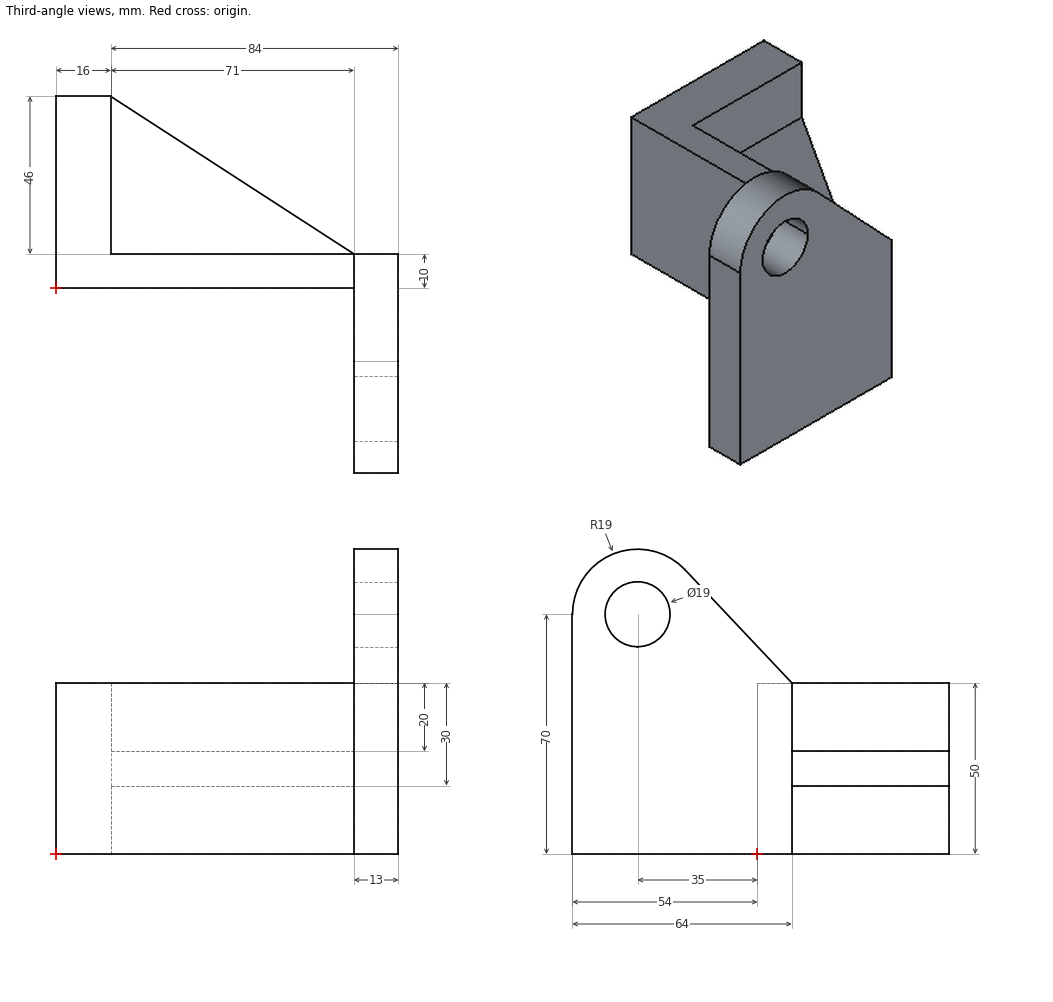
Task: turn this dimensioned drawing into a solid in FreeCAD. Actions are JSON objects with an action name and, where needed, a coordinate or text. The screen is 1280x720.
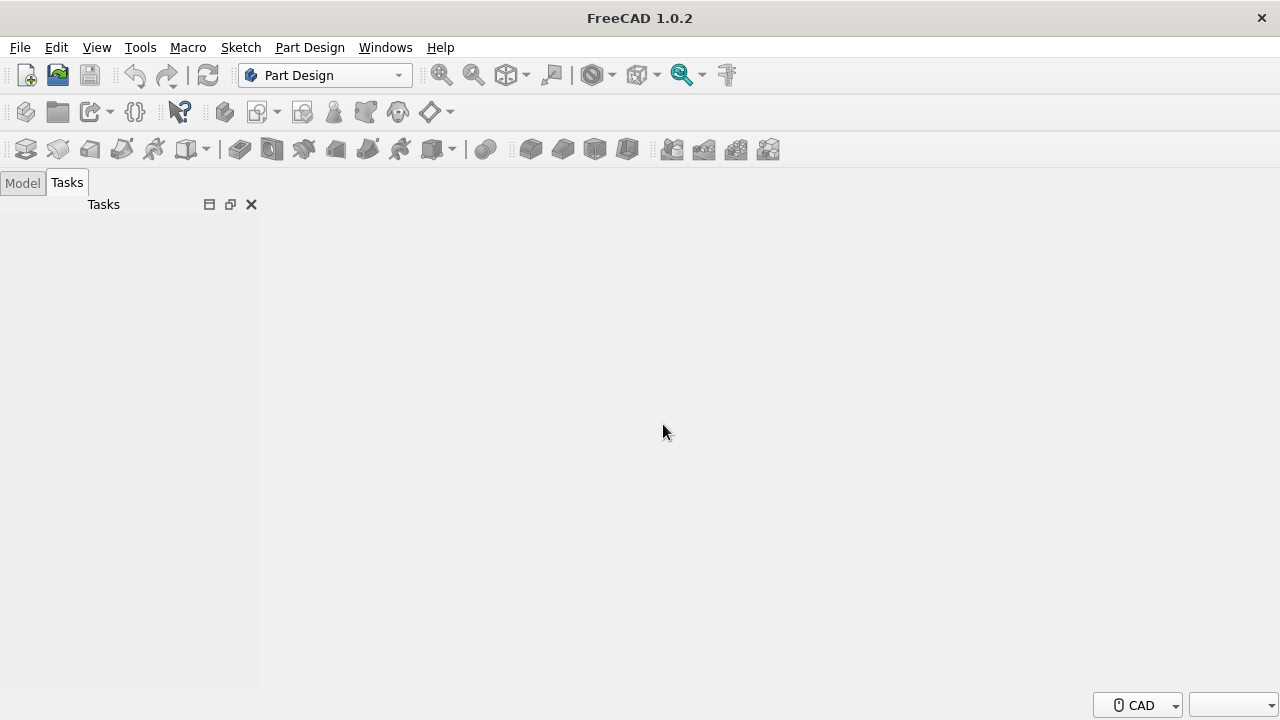
{"action": "key", "text": "ctrl+n"}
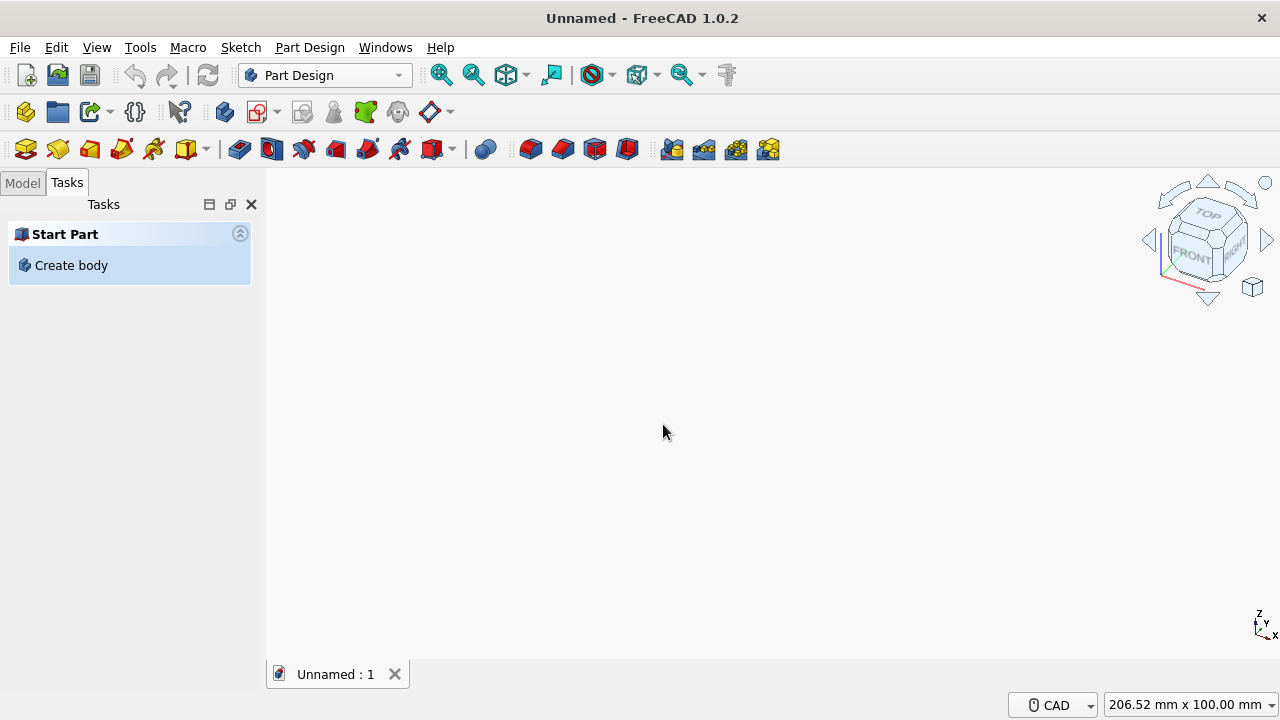
{"action": "left_click", "coordinate": [258, 112]}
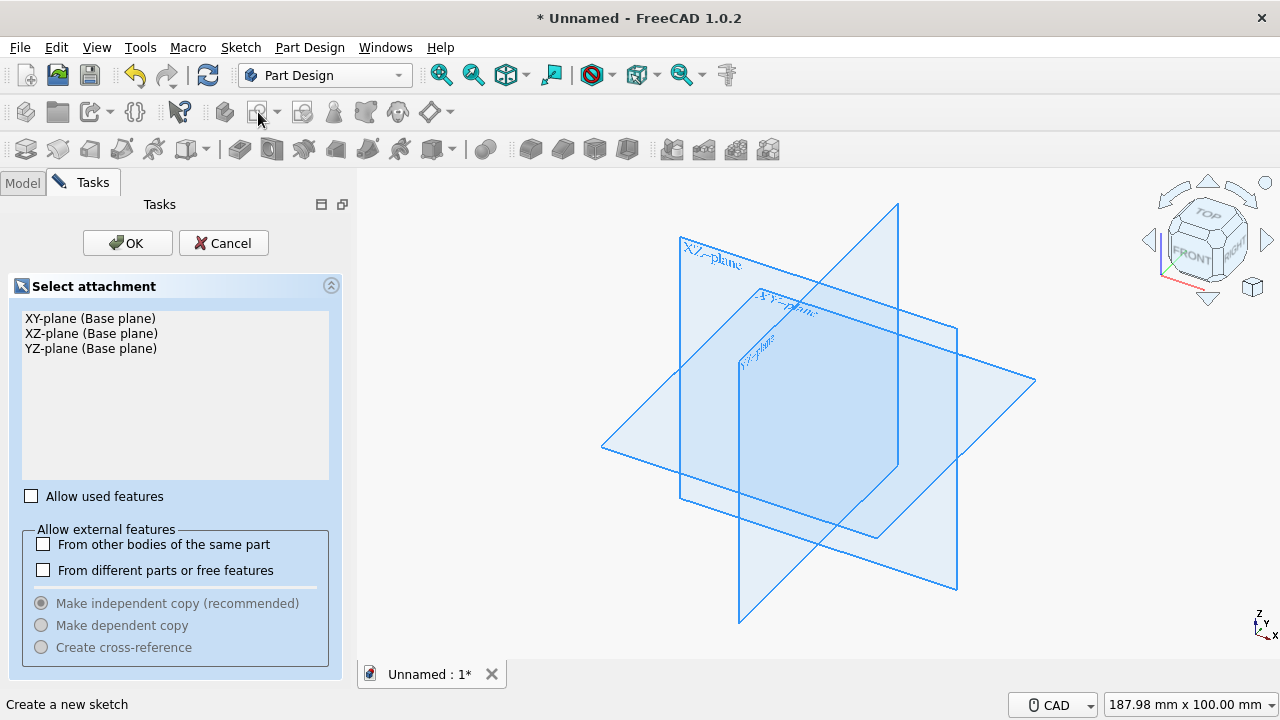
{"action": "left_click", "coordinate": [82, 318]}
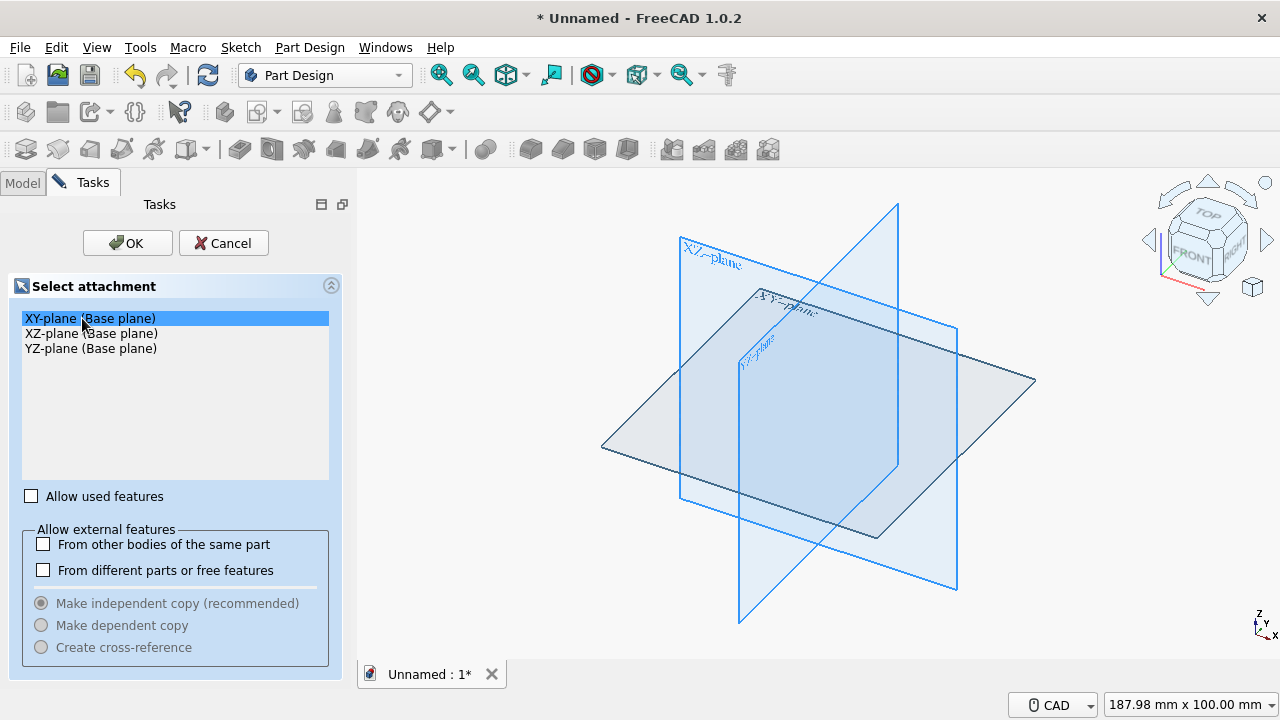
{"action": "left_click", "coordinate": [128, 243]}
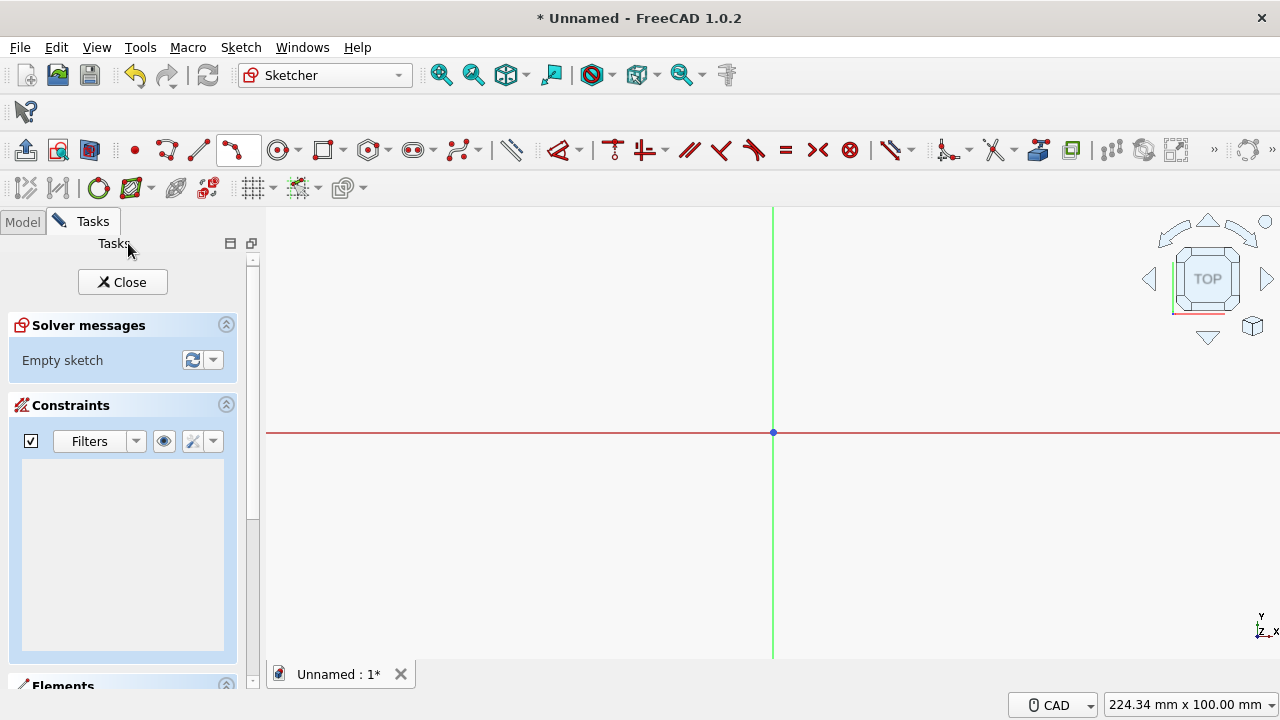
{"action": "scroll", "coordinate": [294, 631], "scroll_direction": "down", "scroll_amount": 1}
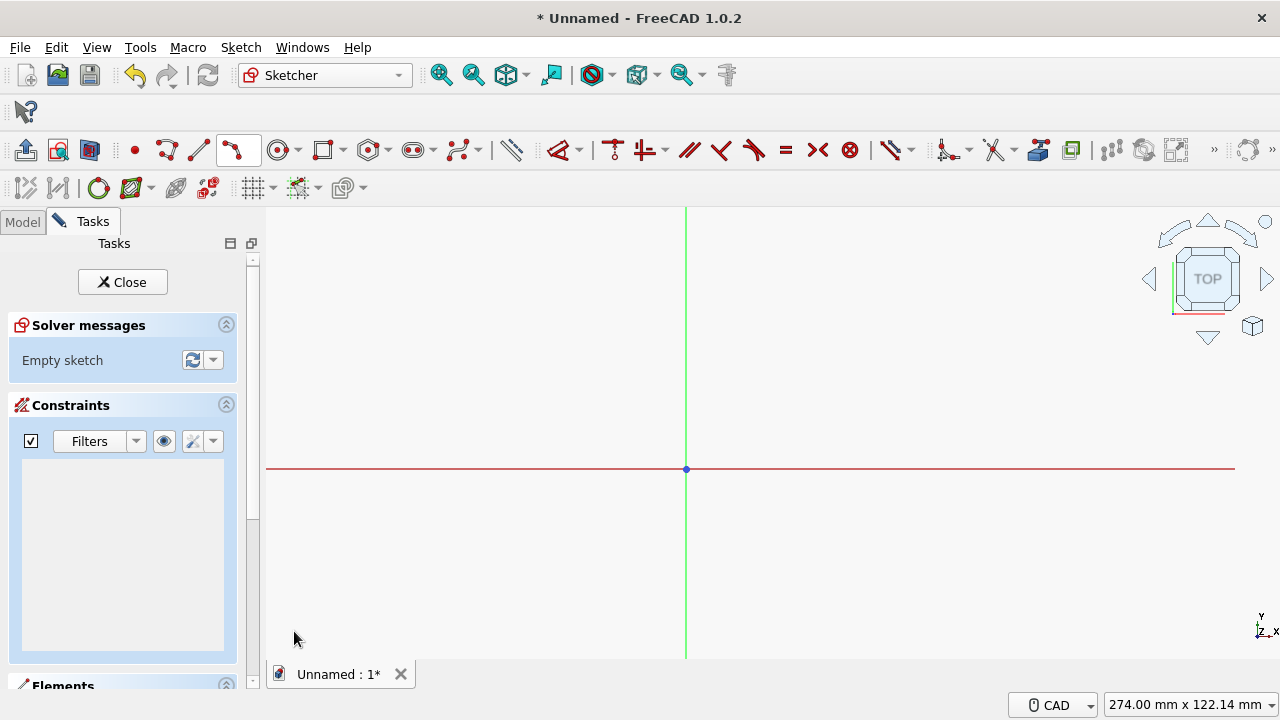
{"action": "key", "text": "g m"}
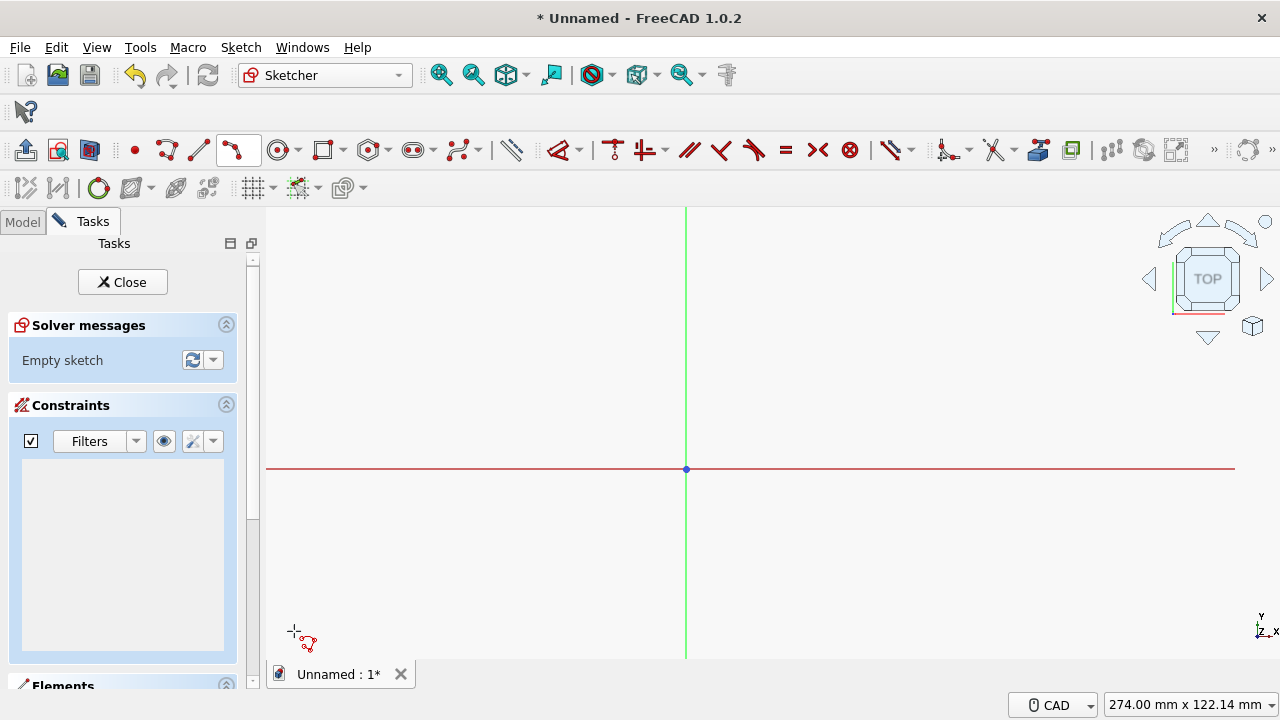
{"action": "left_click", "coordinate": [686, 469]}
{"action": "left_click", "coordinate": [1056, 460]}
{"action": "left_click", "coordinate": [1056, 432]}
{"action": "left_click", "coordinate": [745, 432]}
{"action": "left_click", "coordinate": [745, 262]}
{"action": "left_click", "coordinate": [695, 262]}
{"action": "left_click", "coordinate": [686, 469]}
{"action": "key", "text": "Escape"}
{"action": "key", "text": "Escape"}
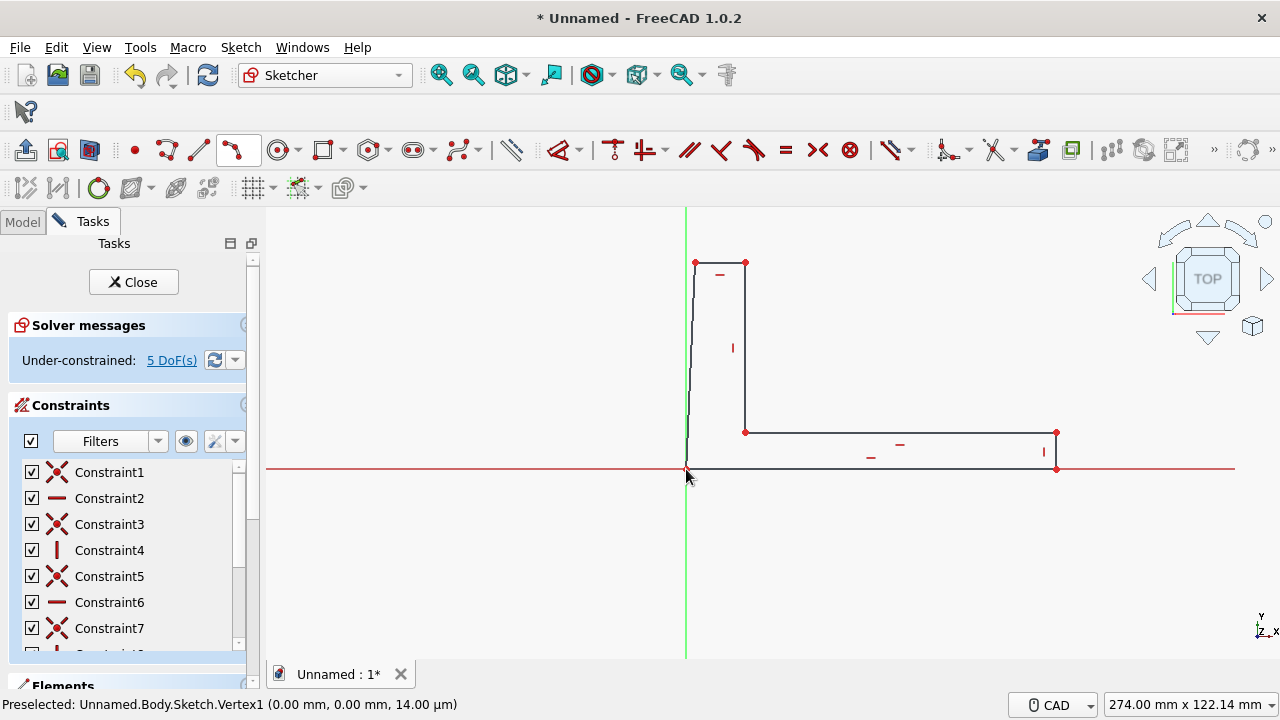
{"action": "left_click", "coordinate": [689, 407]}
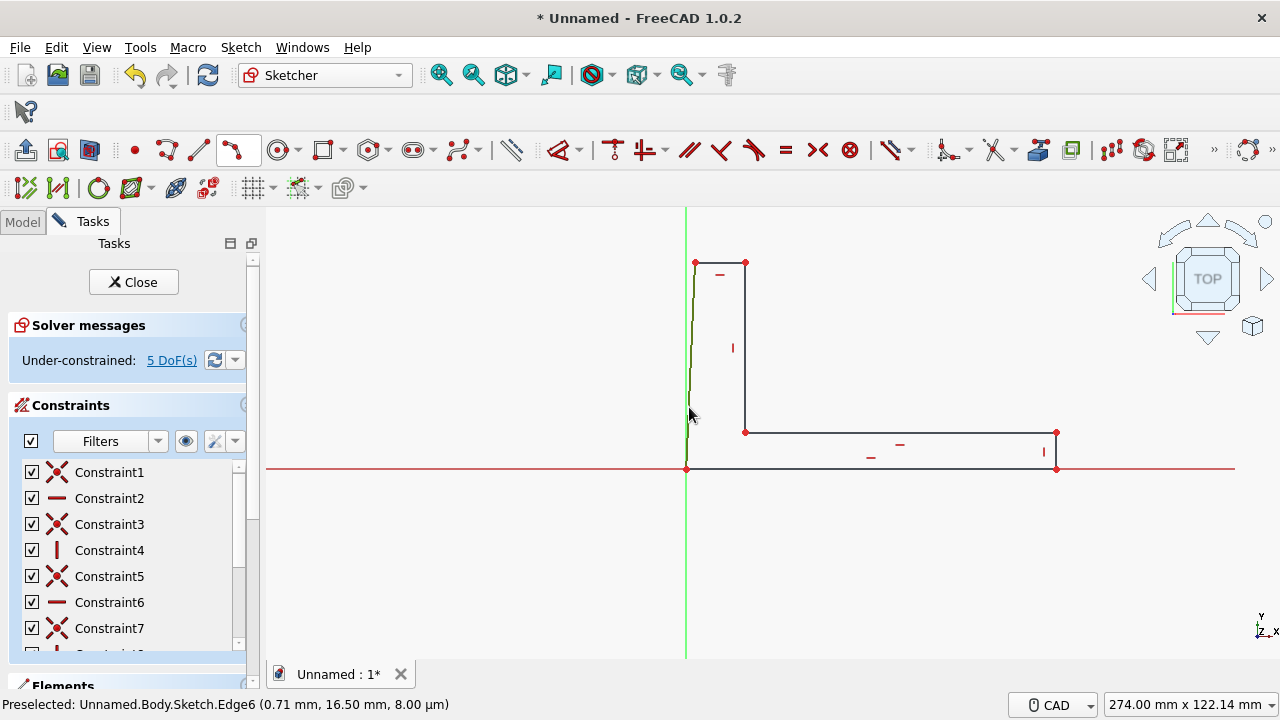
{"action": "left_click", "coordinate": [668, 150]}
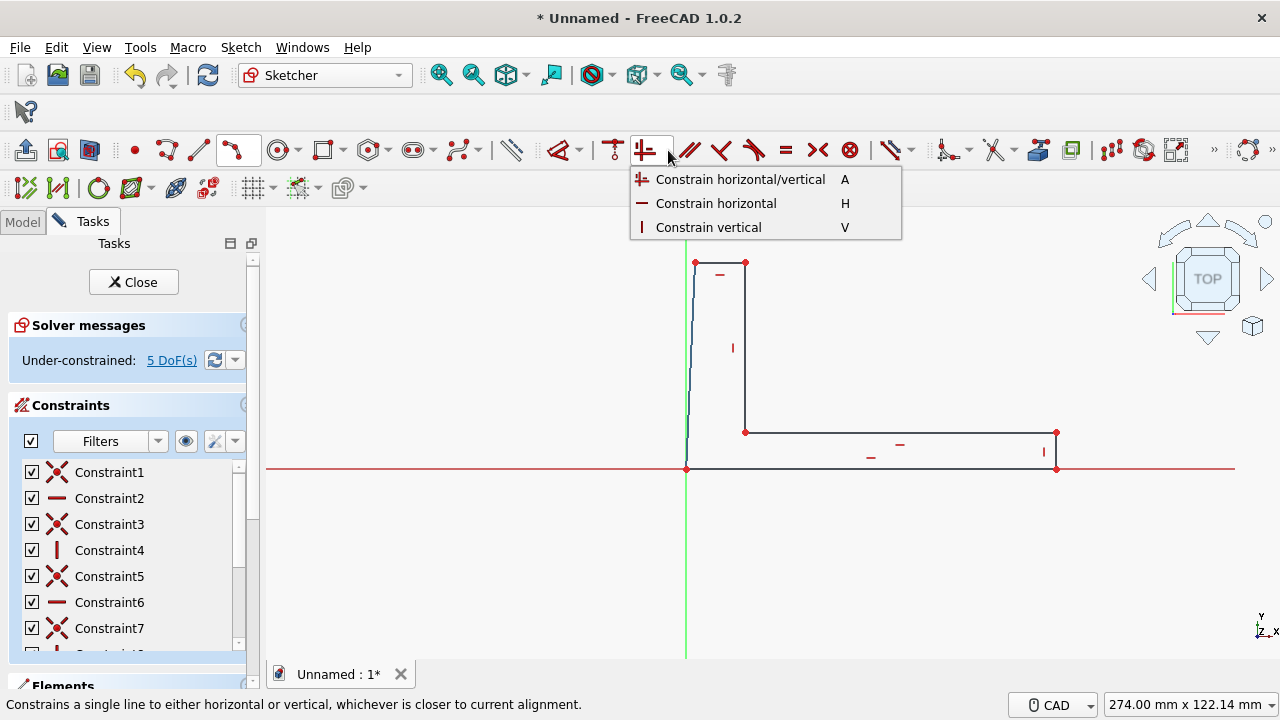
{"action": "left_click", "coordinate": [766, 227]}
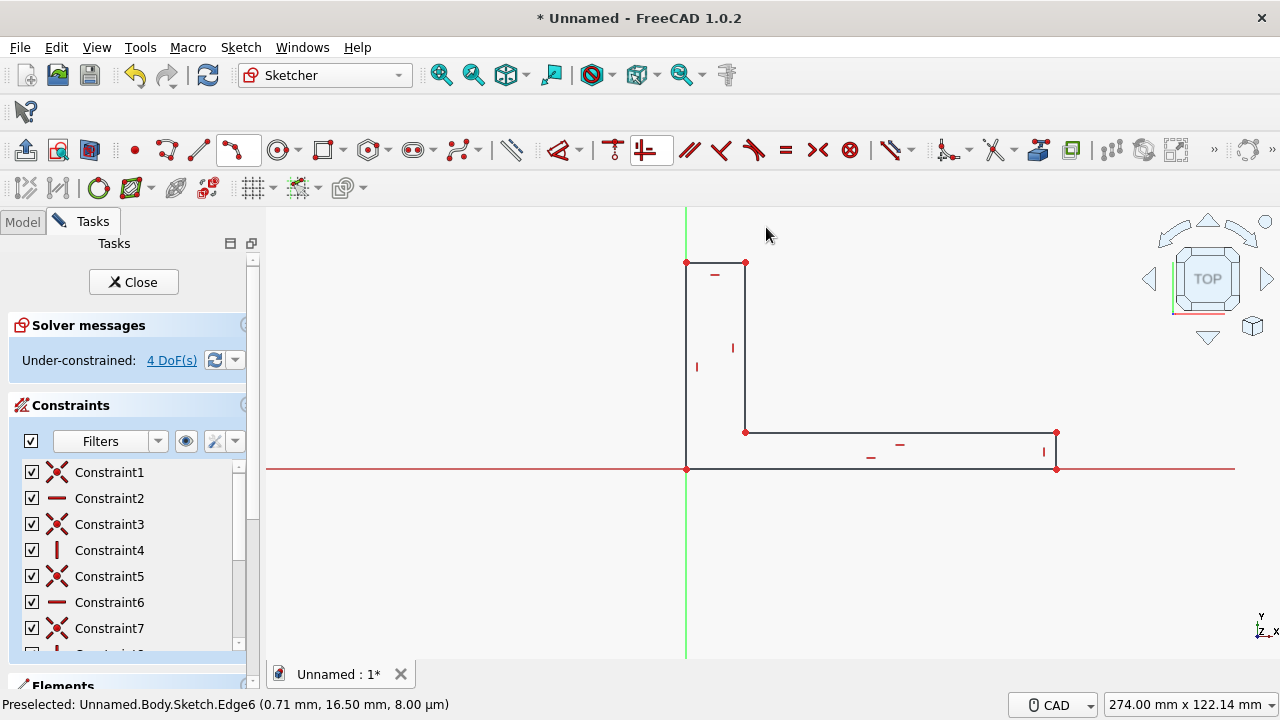
{"action": "key", "text": "d"}